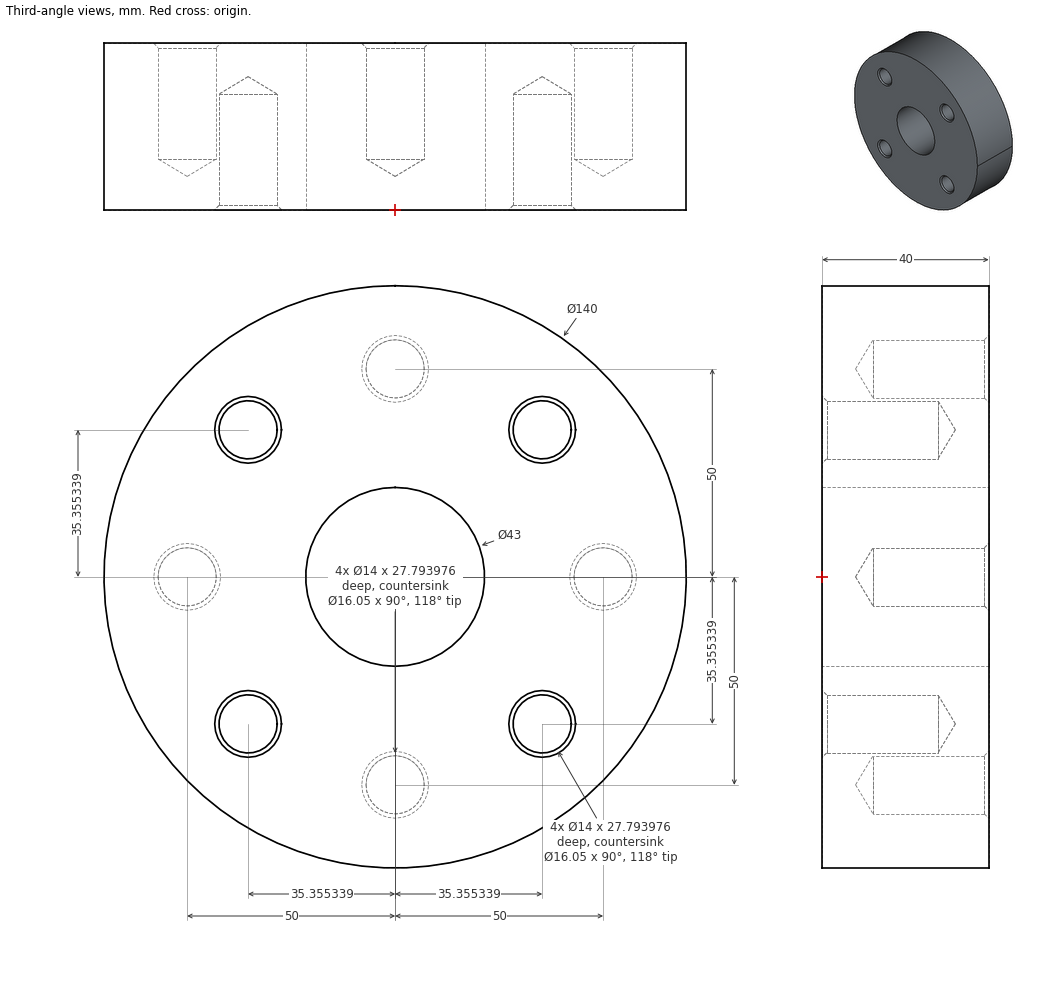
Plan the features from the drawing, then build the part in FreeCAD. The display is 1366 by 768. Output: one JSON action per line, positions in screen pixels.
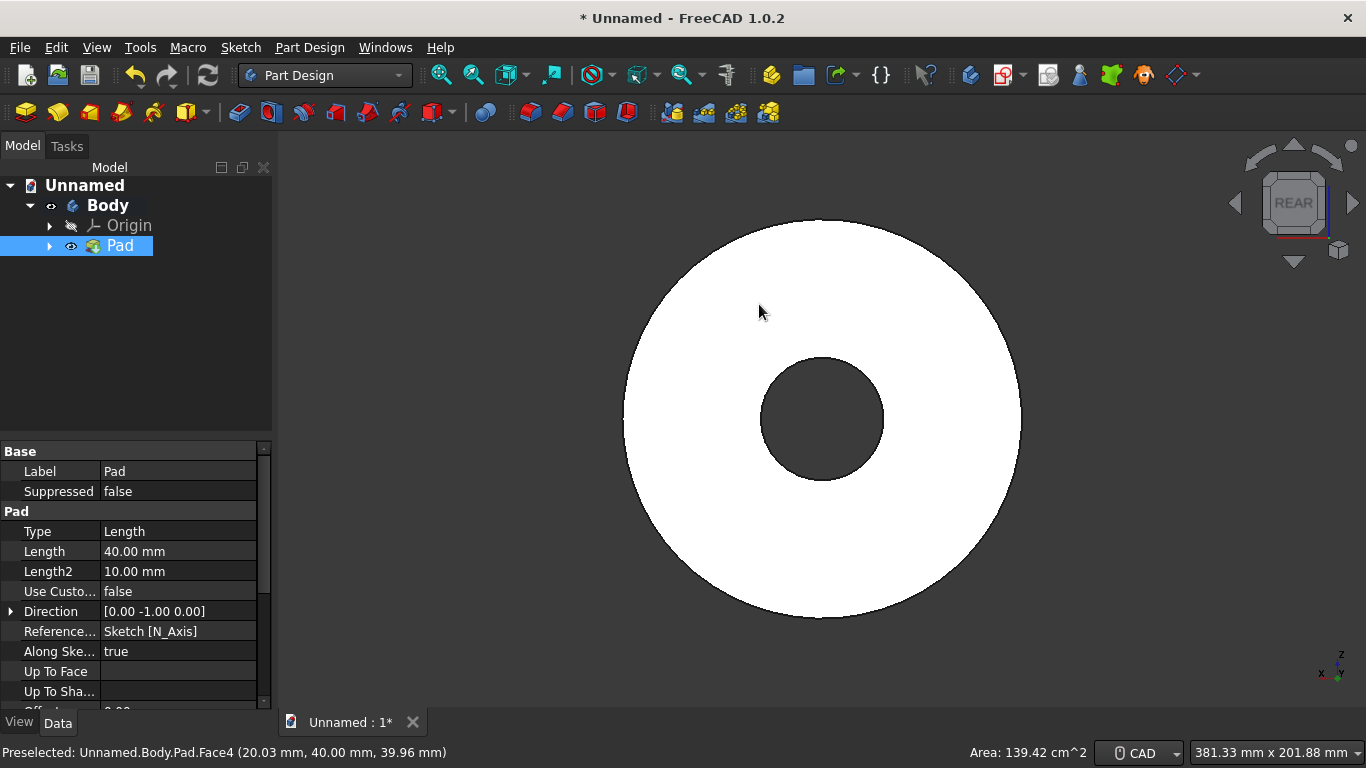
{"action": "left_click", "coordinate": [1004, 76]}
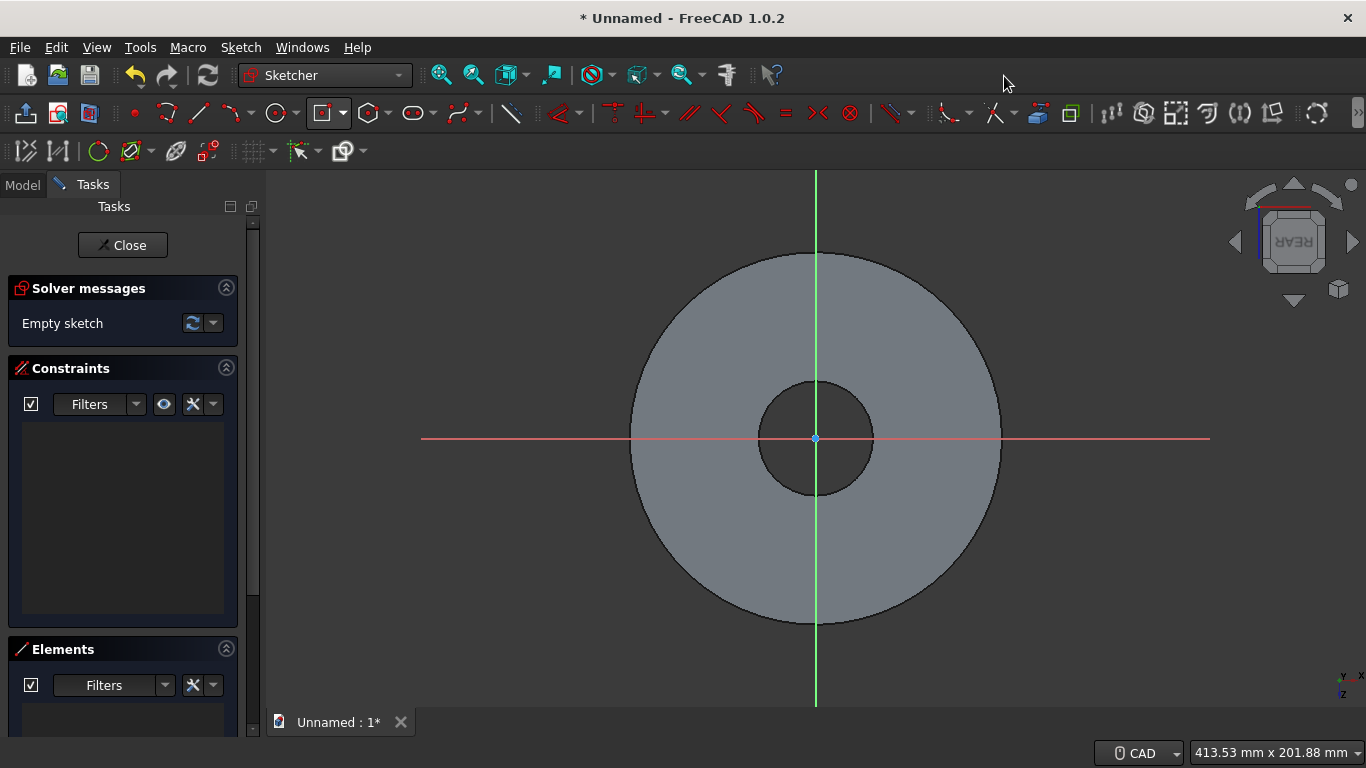
{"action": "left_click", "coordinate": [276, 114]}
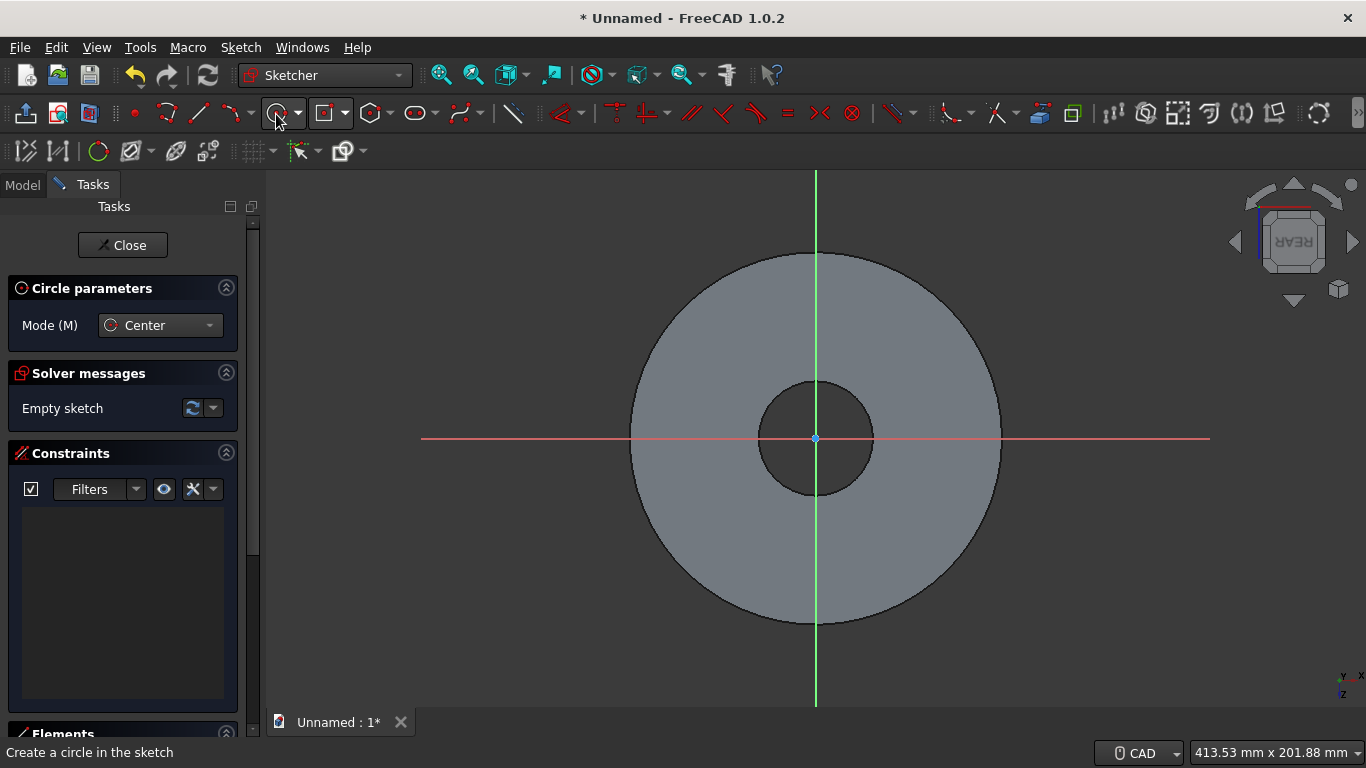
{"action": "left_click", "coordinate": [816, 305]}
{"action": "mouse_move", "coordinate": [833, 299]}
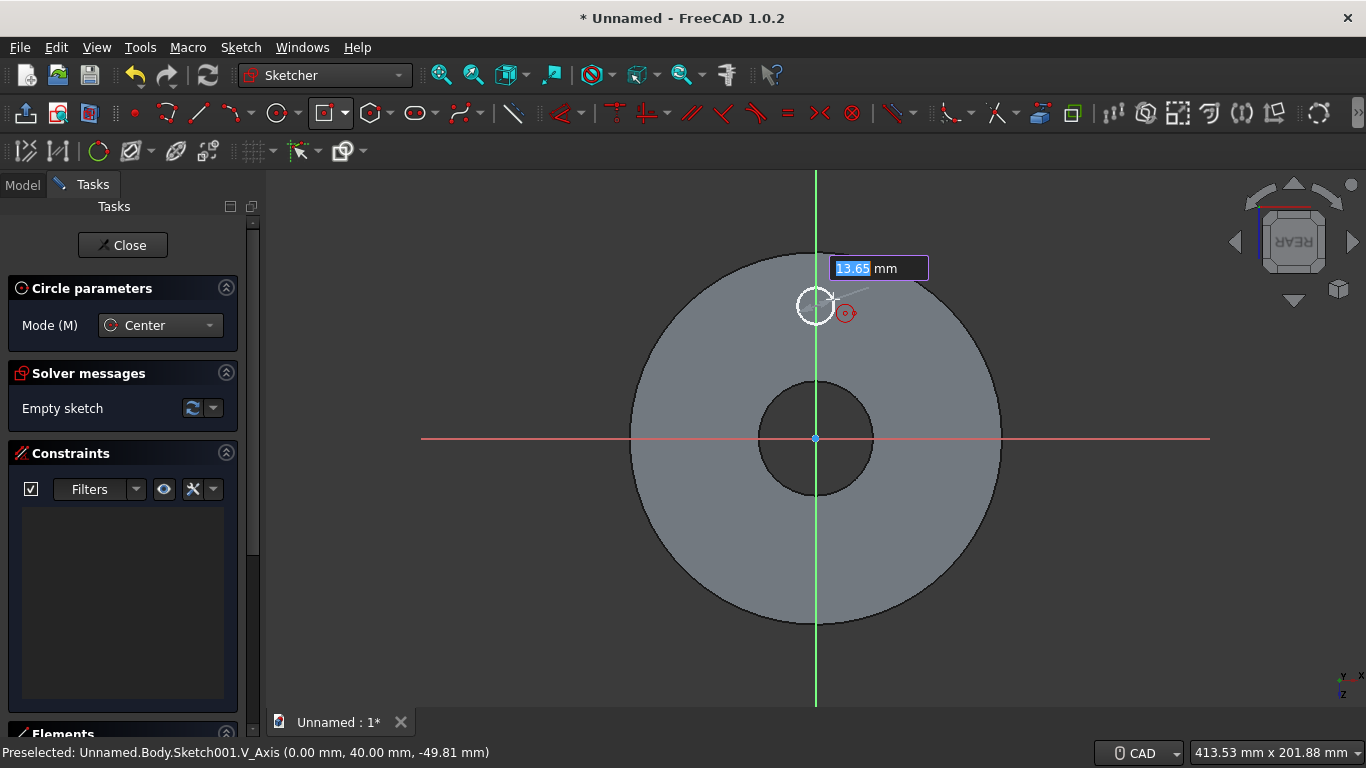
{"action": "type", "text": "14"}
{"action": "key", "text": "Return"}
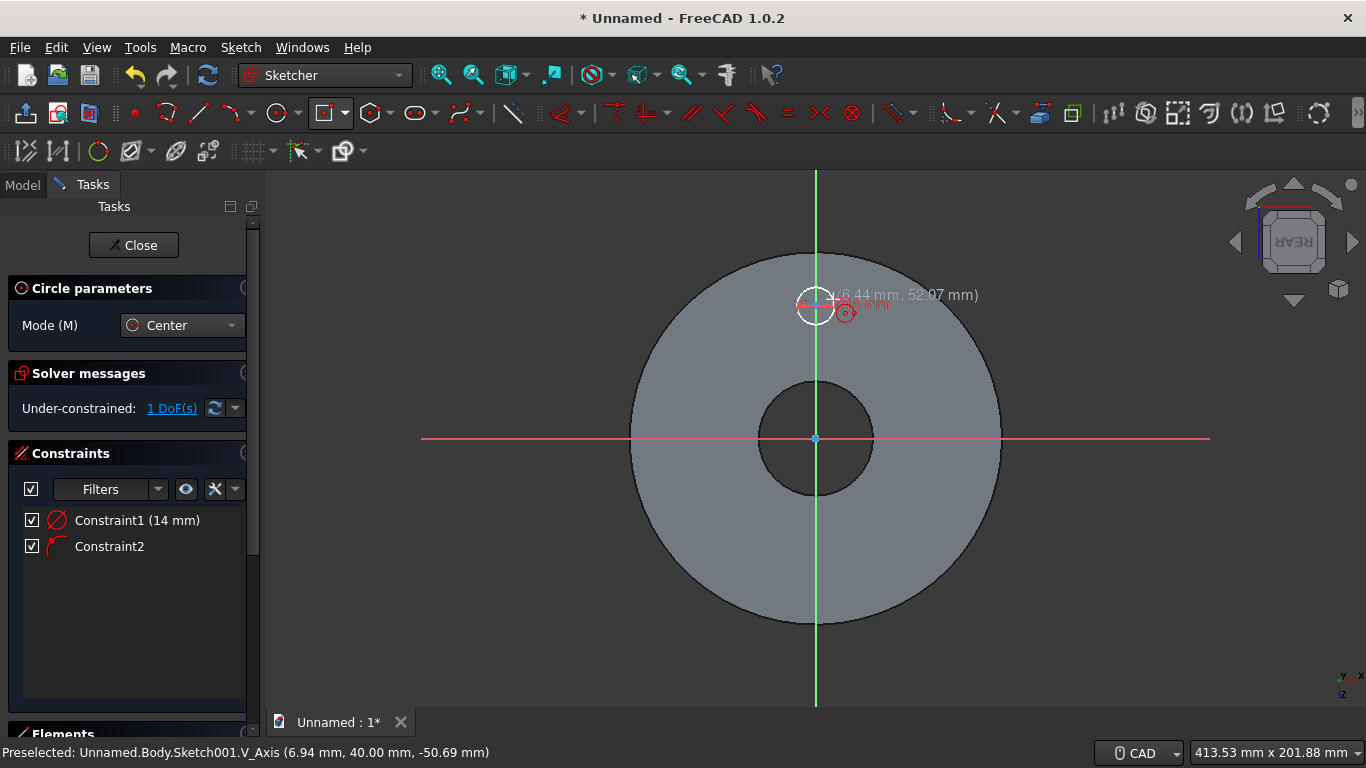
{"action": "left_click", "coordinate": [949, 439]}
{"action": "mouse_move", "coordinate": [955, 421]}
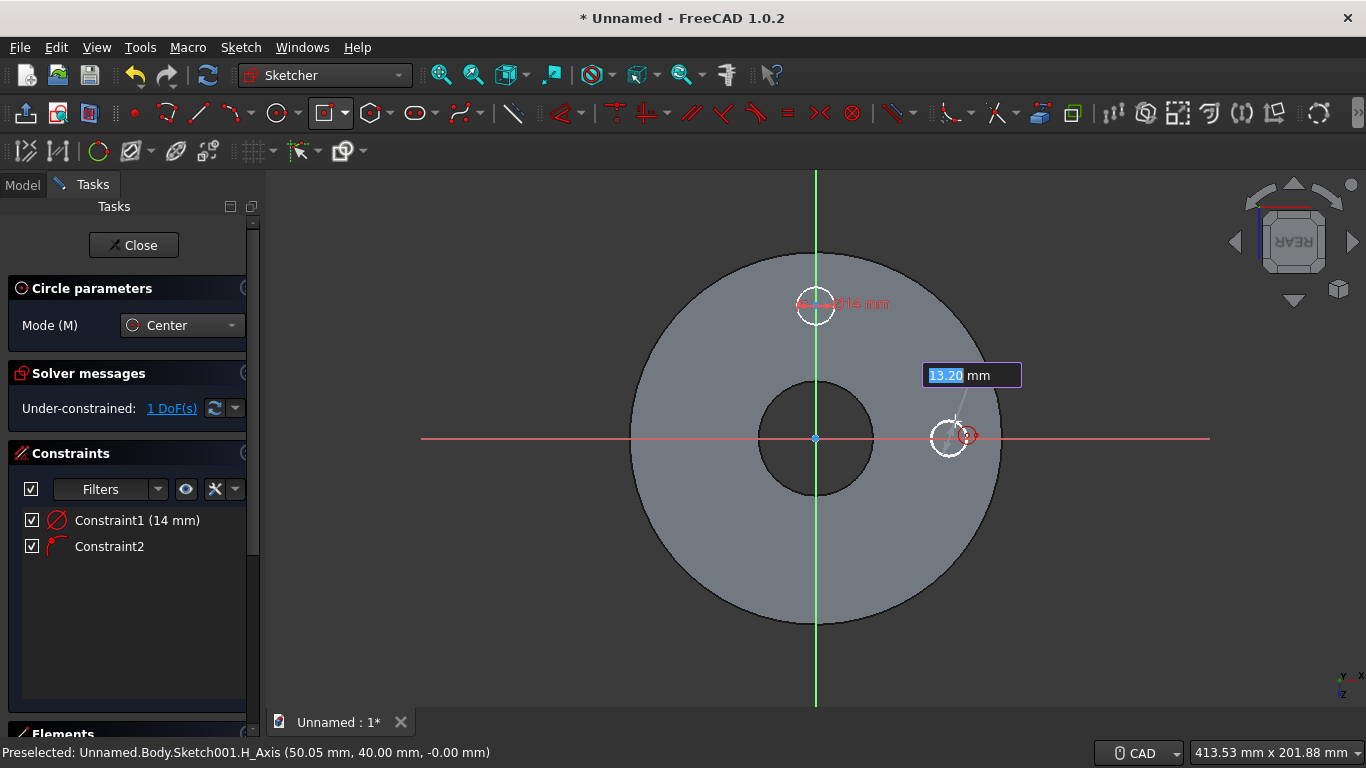
{"action": "type", "text": "14"}
{"action": "key", "text": "Return"}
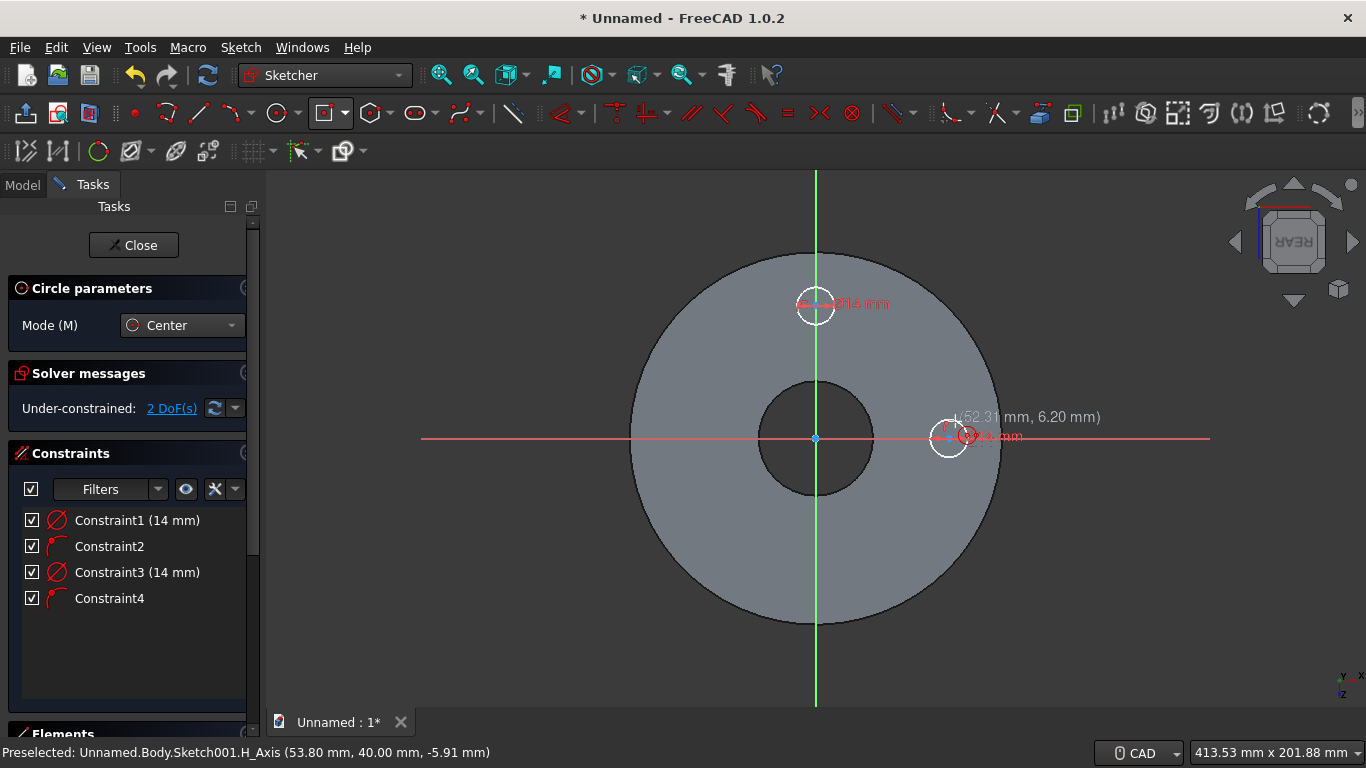
{"action": "left_click", "coordinate": [816, 572]}
{"action": "mouse_move", "coordinate": [833, 565]}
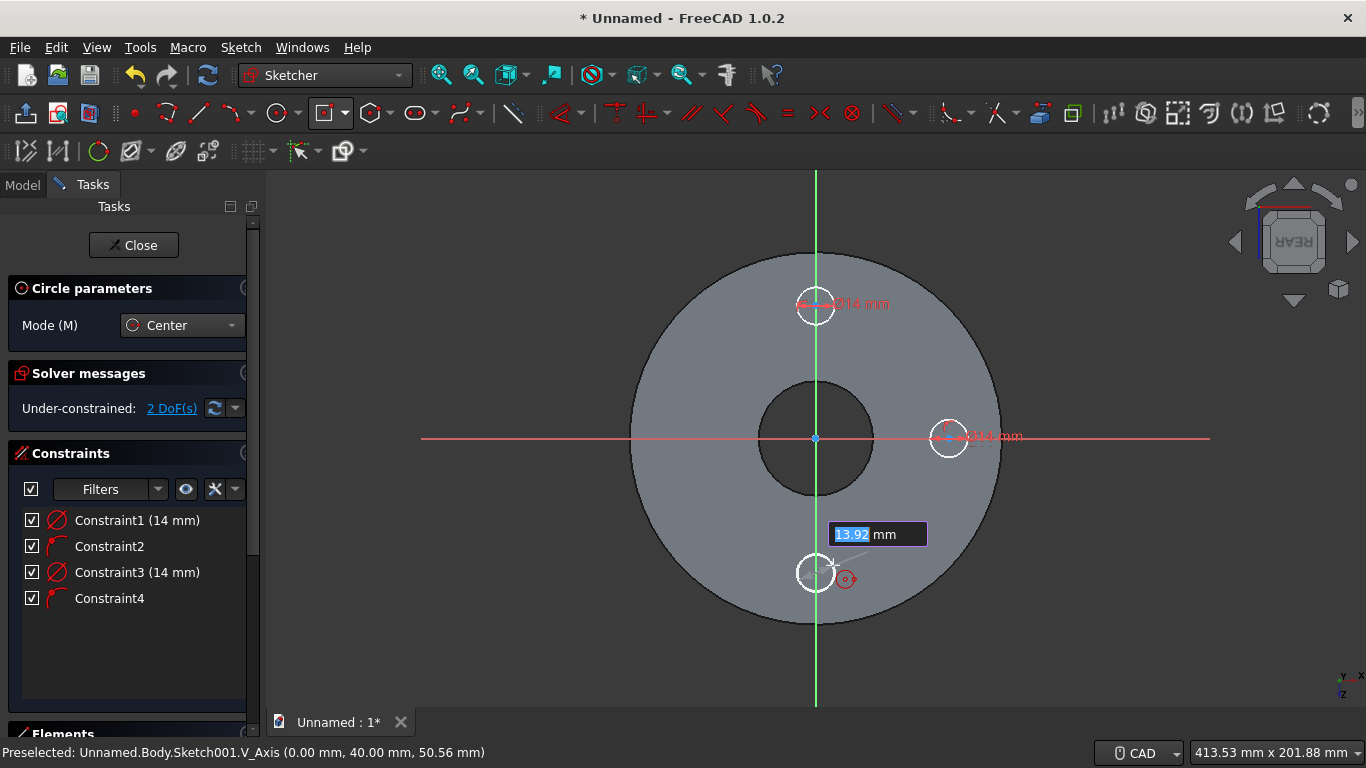
{"action": "type", "text": "14"}
{"action": "key", "text": "Return"}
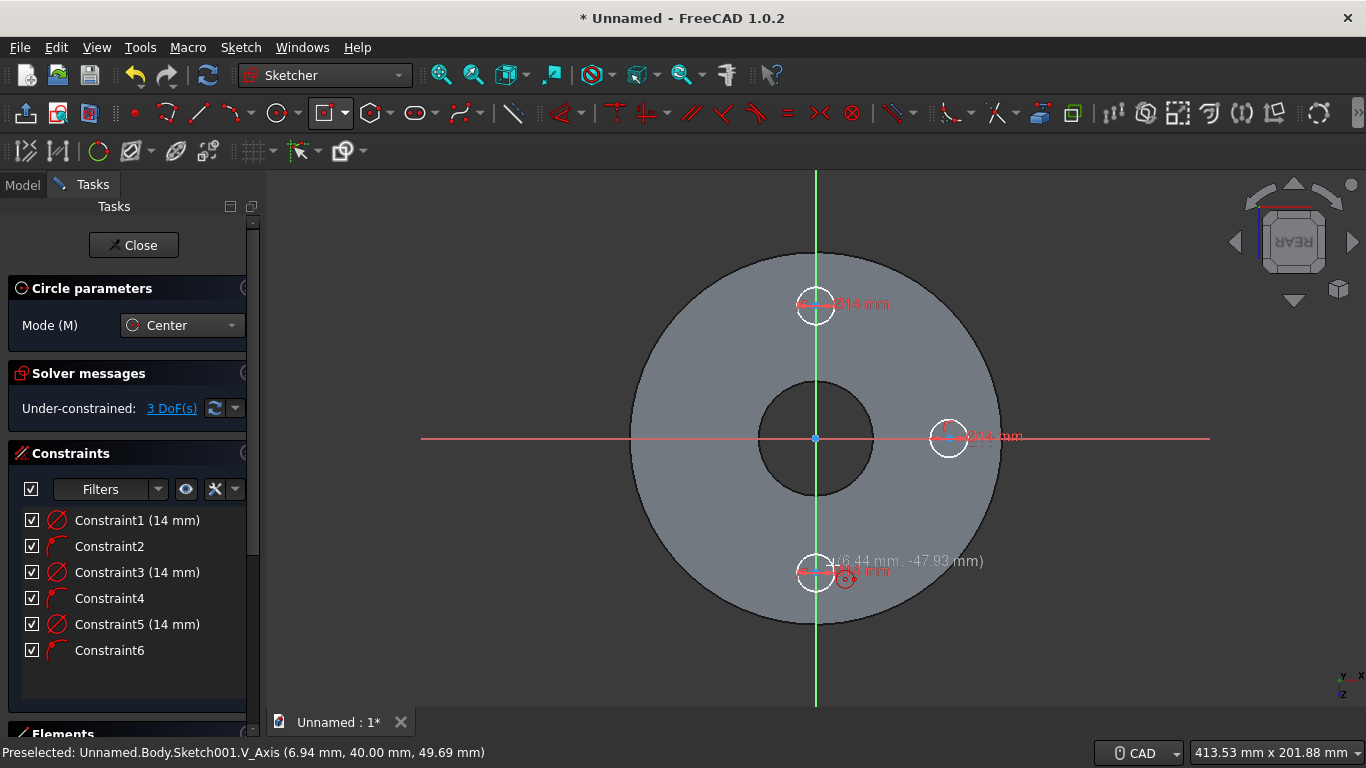
{"action": "left_click", "coordinate": [683, 439]}
{"action": "mouse_move", "coordinate": [689, 421]}